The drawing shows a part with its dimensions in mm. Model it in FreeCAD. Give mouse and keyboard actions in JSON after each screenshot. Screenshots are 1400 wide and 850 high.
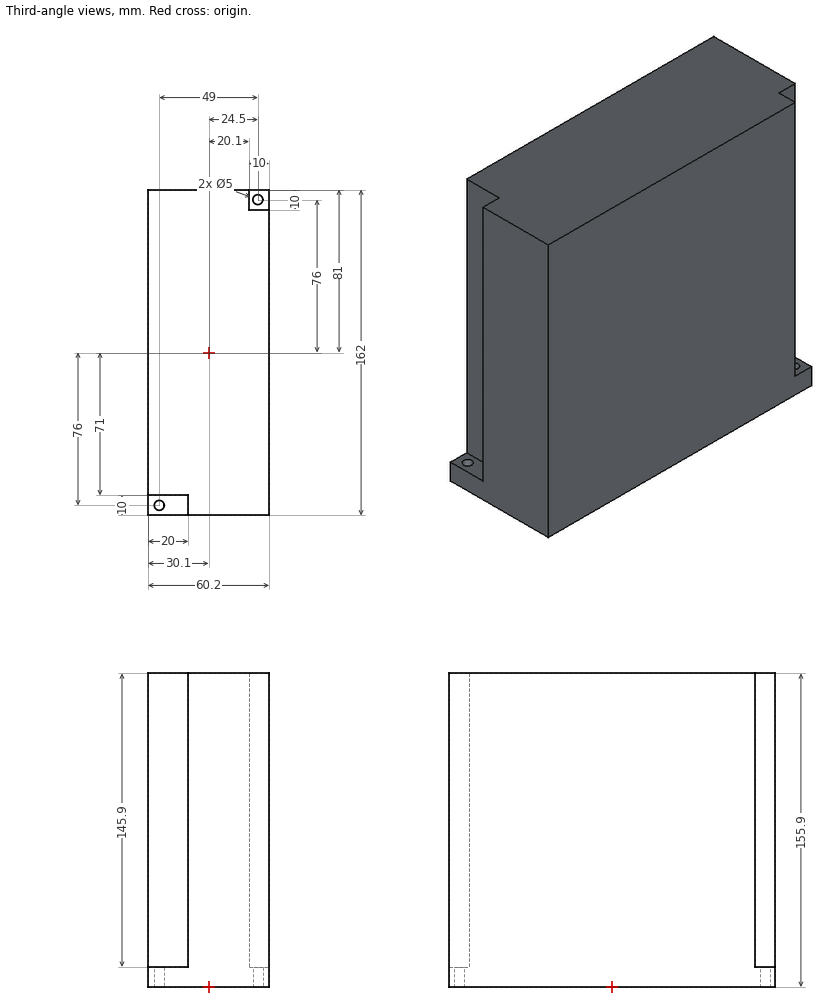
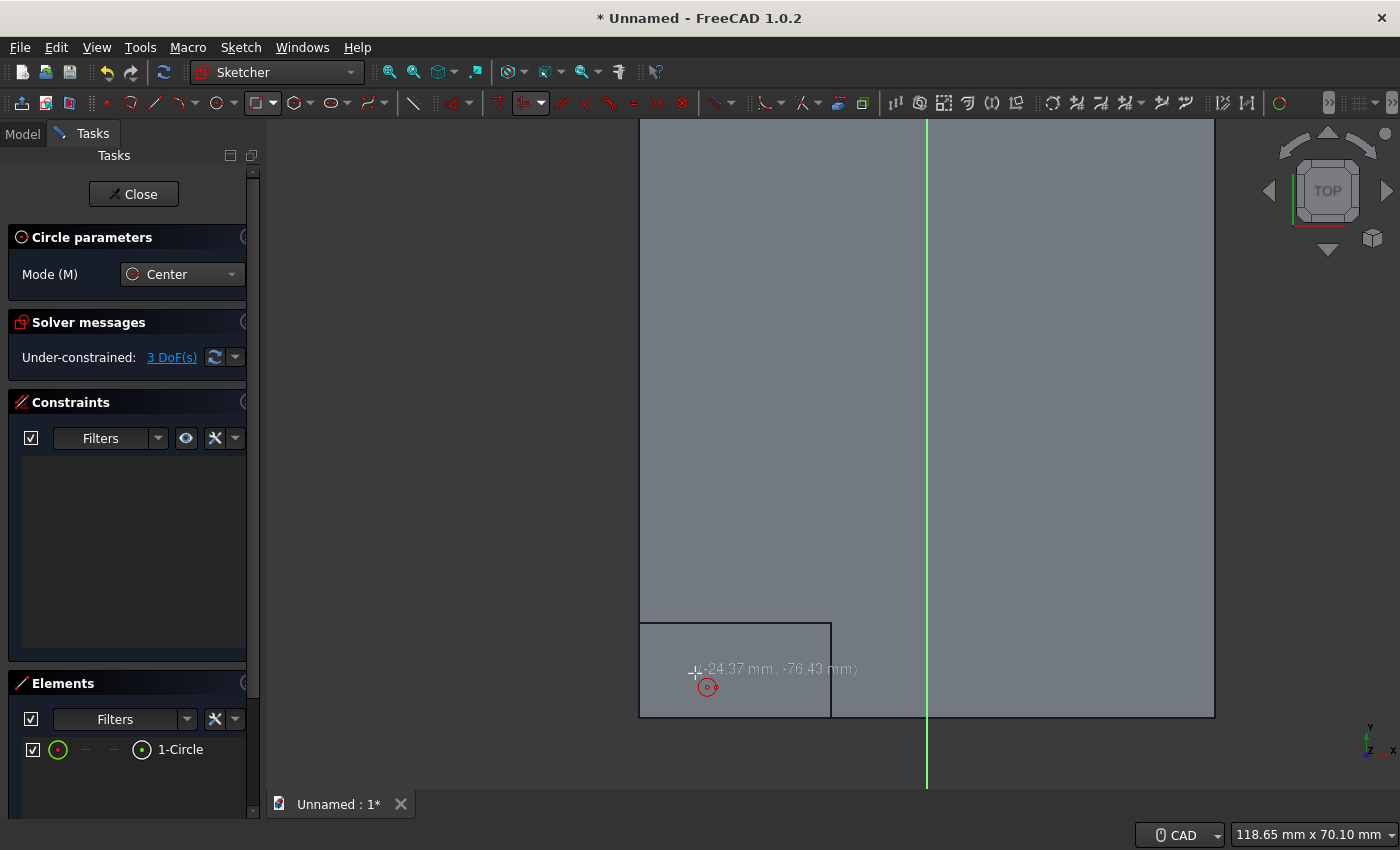
{"action": "left_click", "coordinate": [693, 670]}
{"action": "left_click", "coordinate": [710, 653]}
{"action": "key", "text": "Escape"}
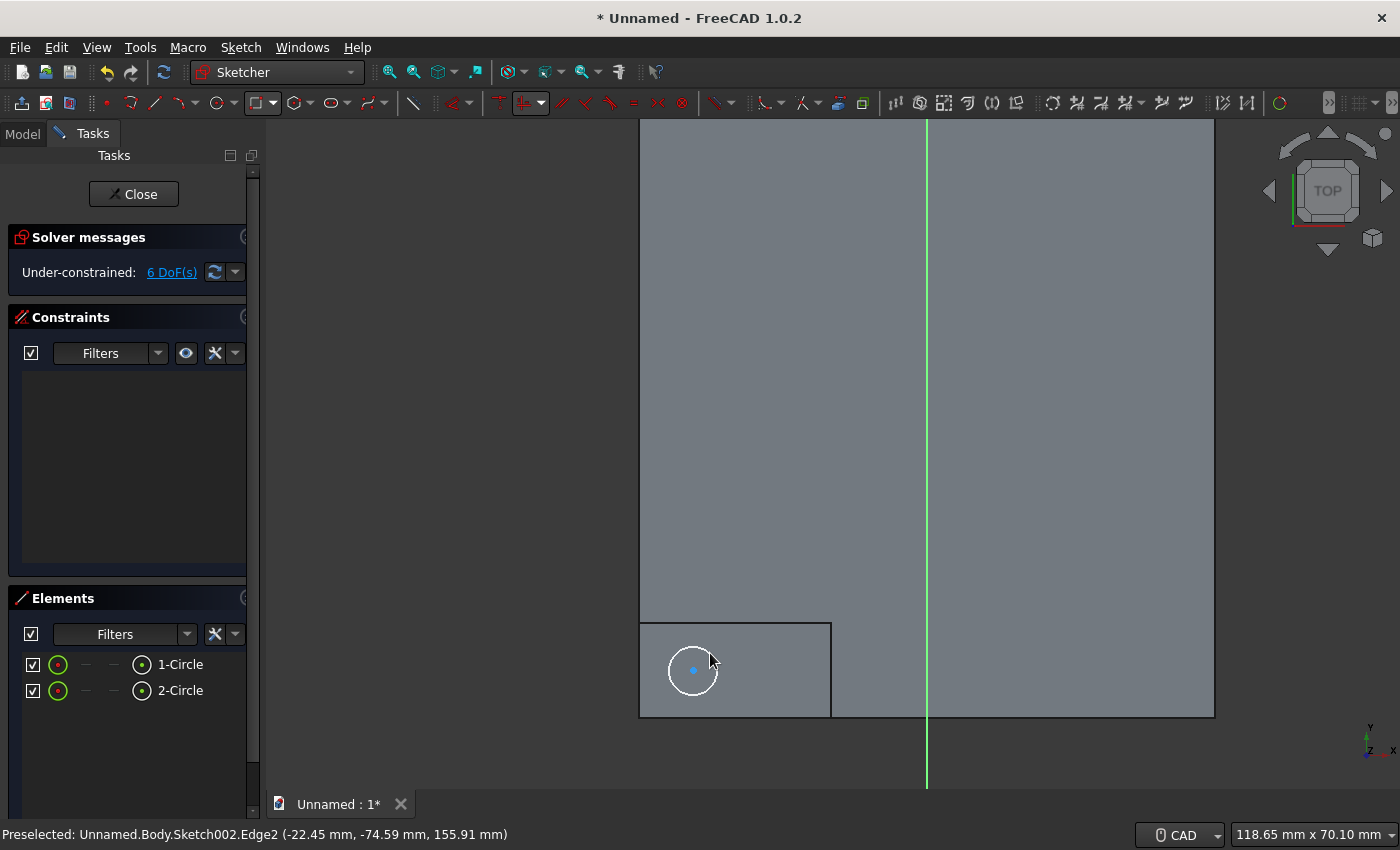
{"action": "scroll", "coordinate": [694, 674], "scroll_direction": "down", "scroll_amount": 6}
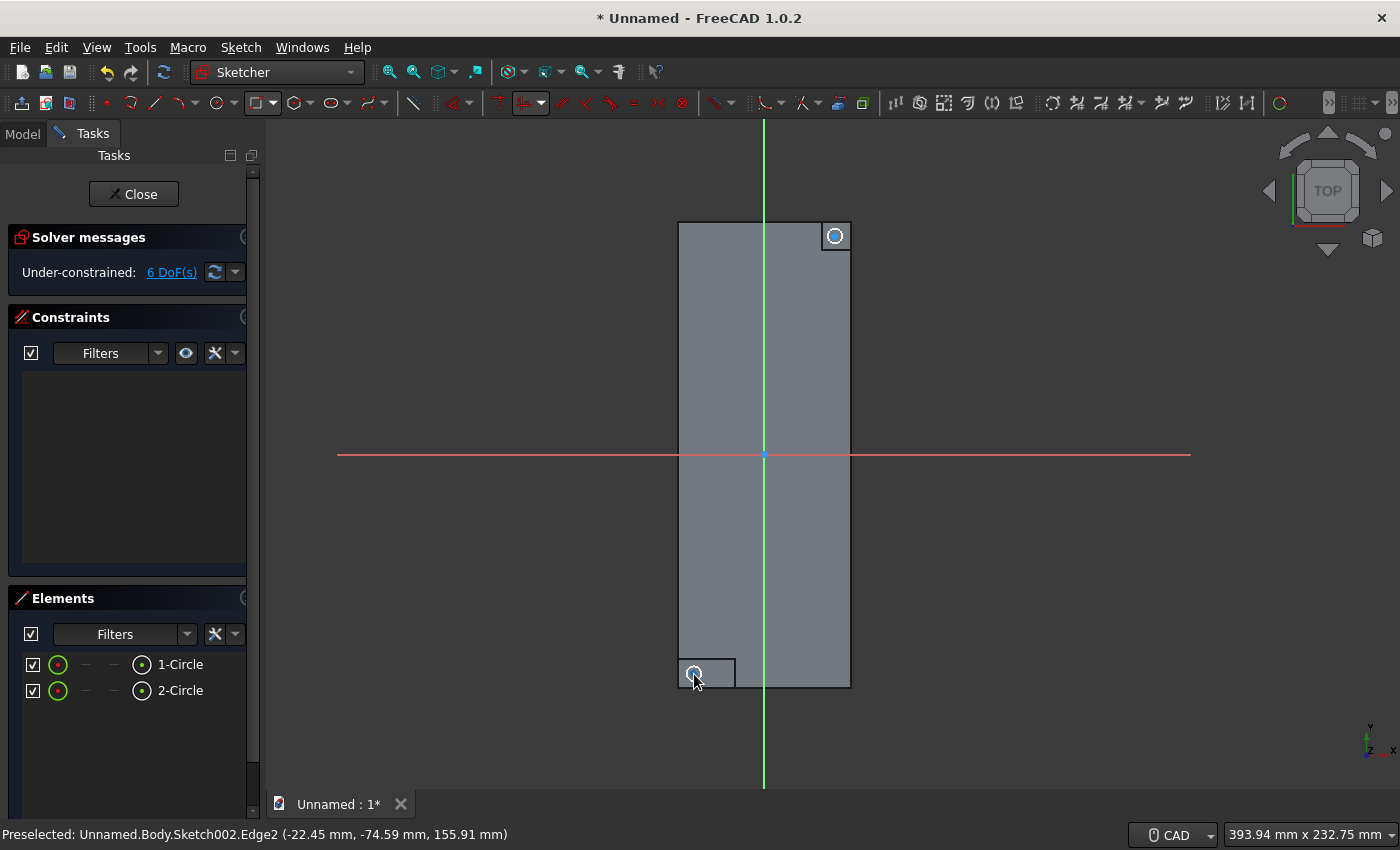
{"action": "scroll", "coordinate": [840, 231], "scroll_direction": "up", "scroll_amount": 4}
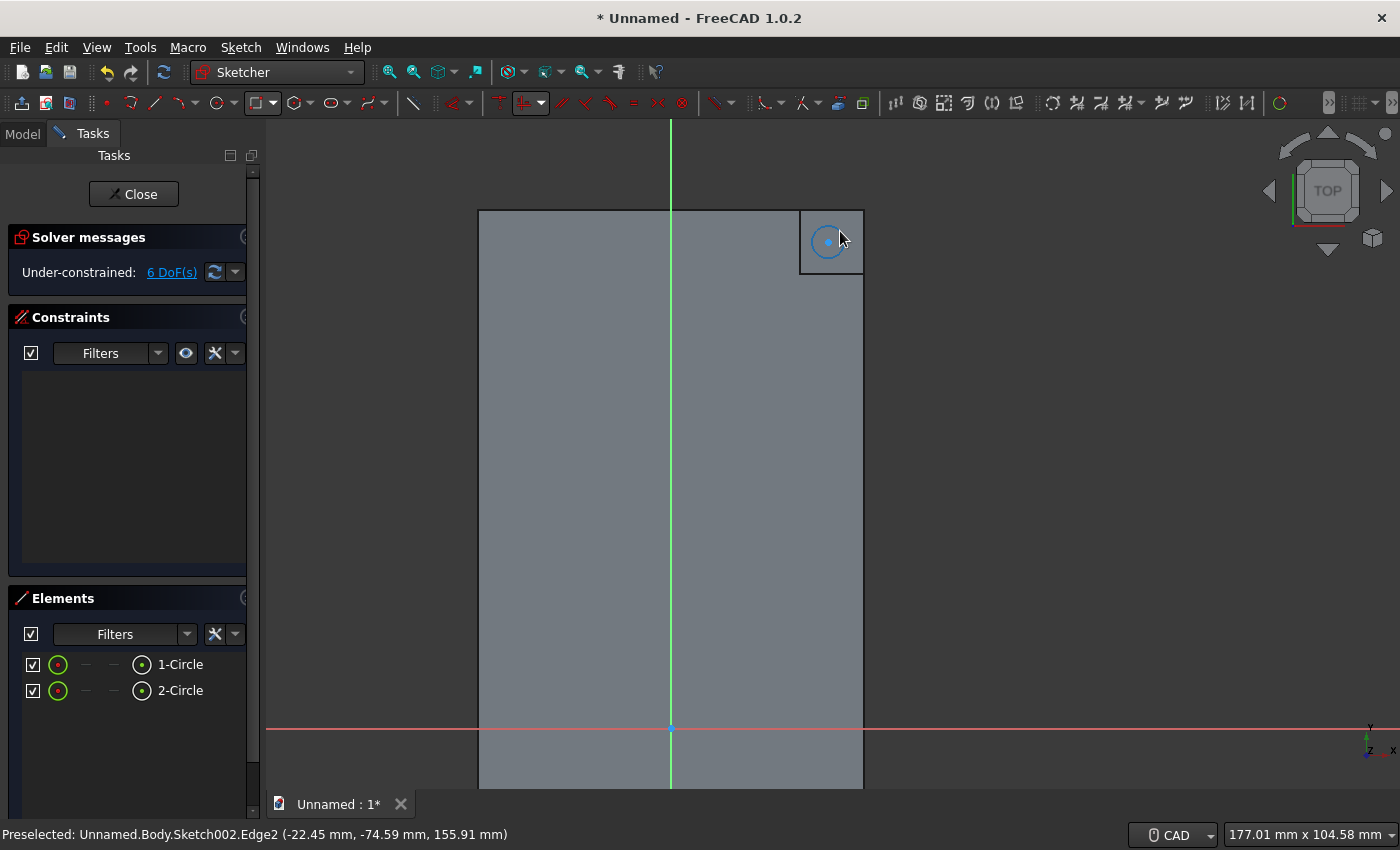
{"action": "left_click", "coordinate": [839, 231]}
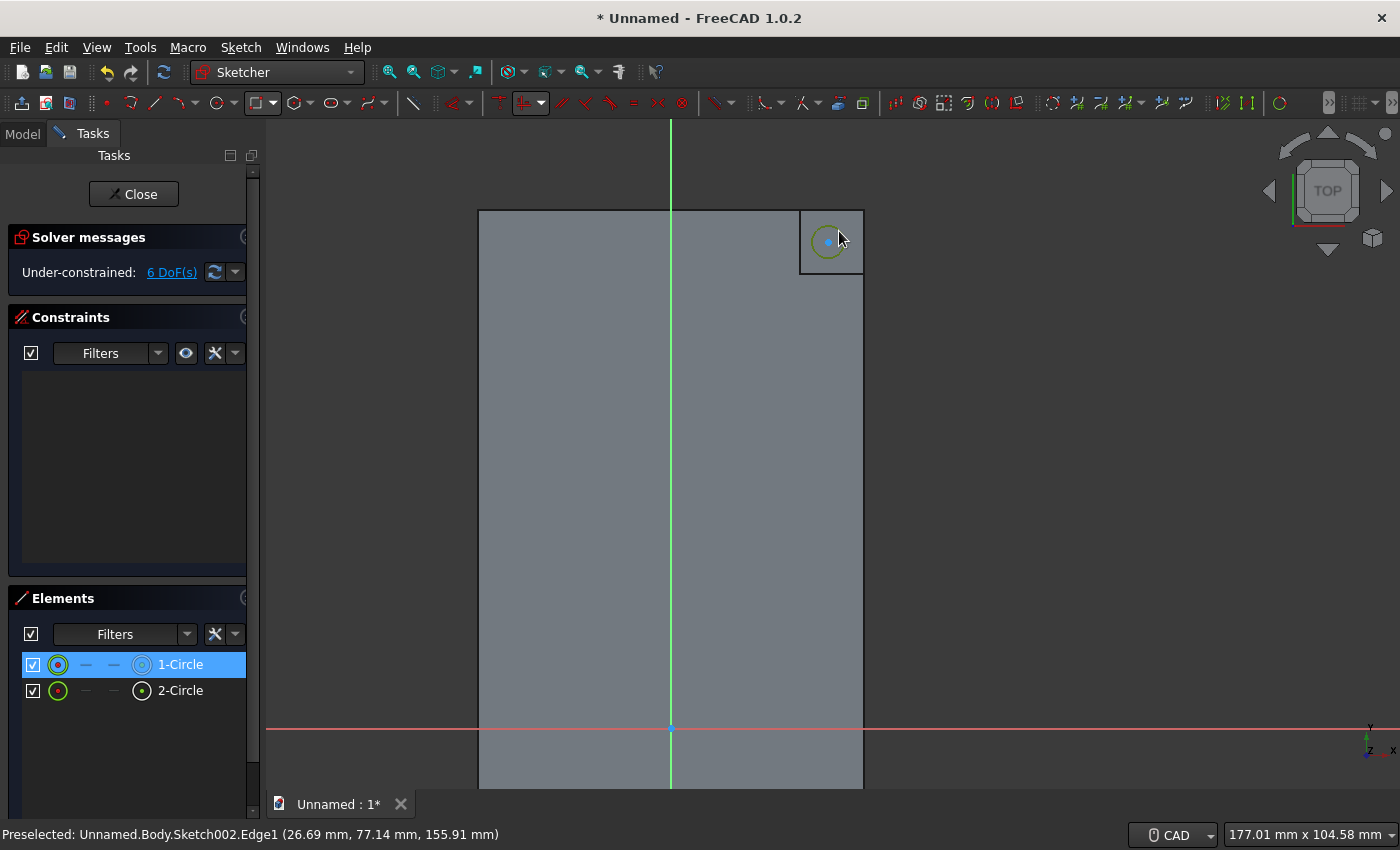
{"action": "scroll", "coordinate": [841, 230], "scroll_direction": "down", "scroll_amount": 4}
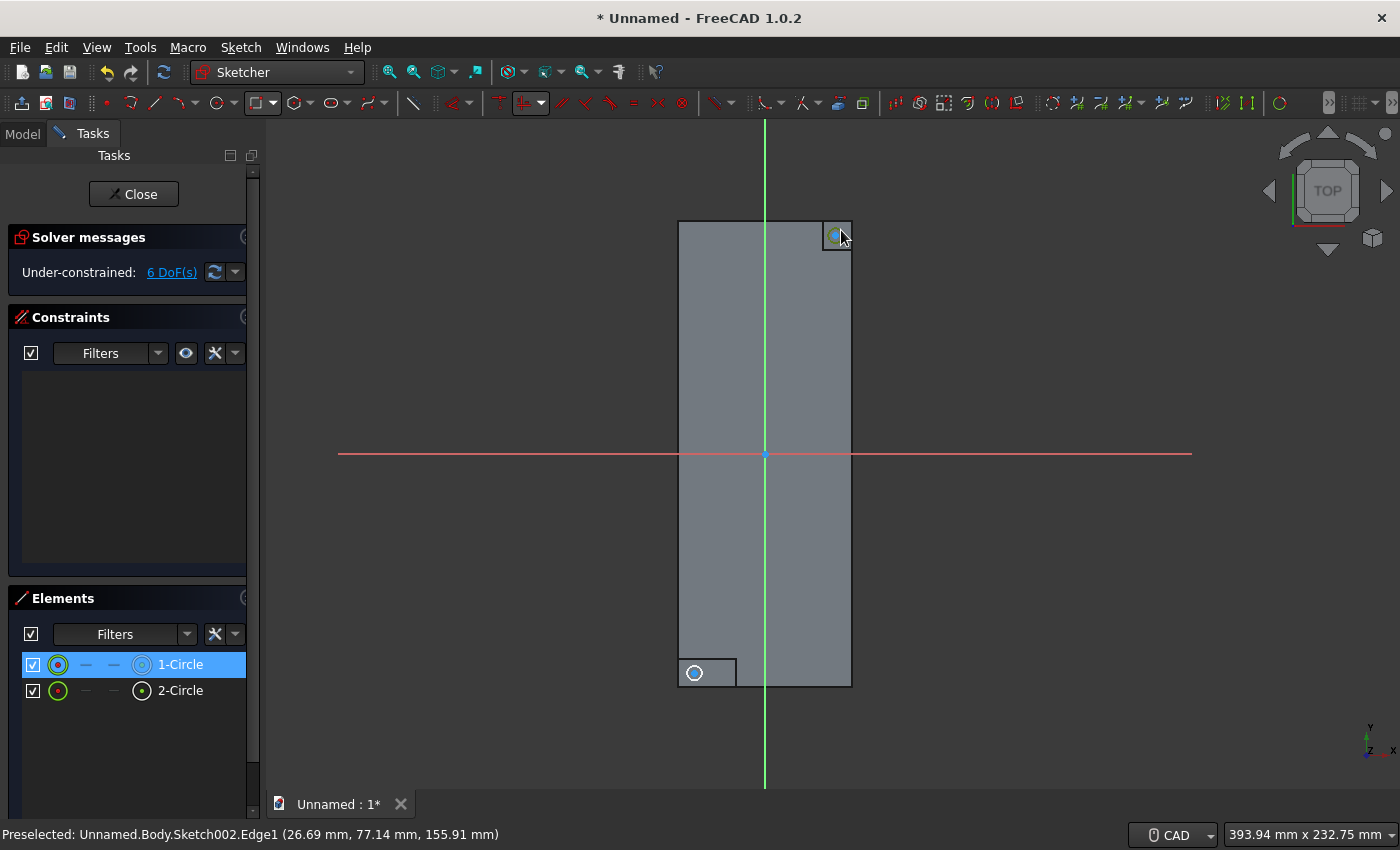
{"action": "scroll", "coordinate": [700, 668], "scroll_direction": "up", "scroll_amount": 4}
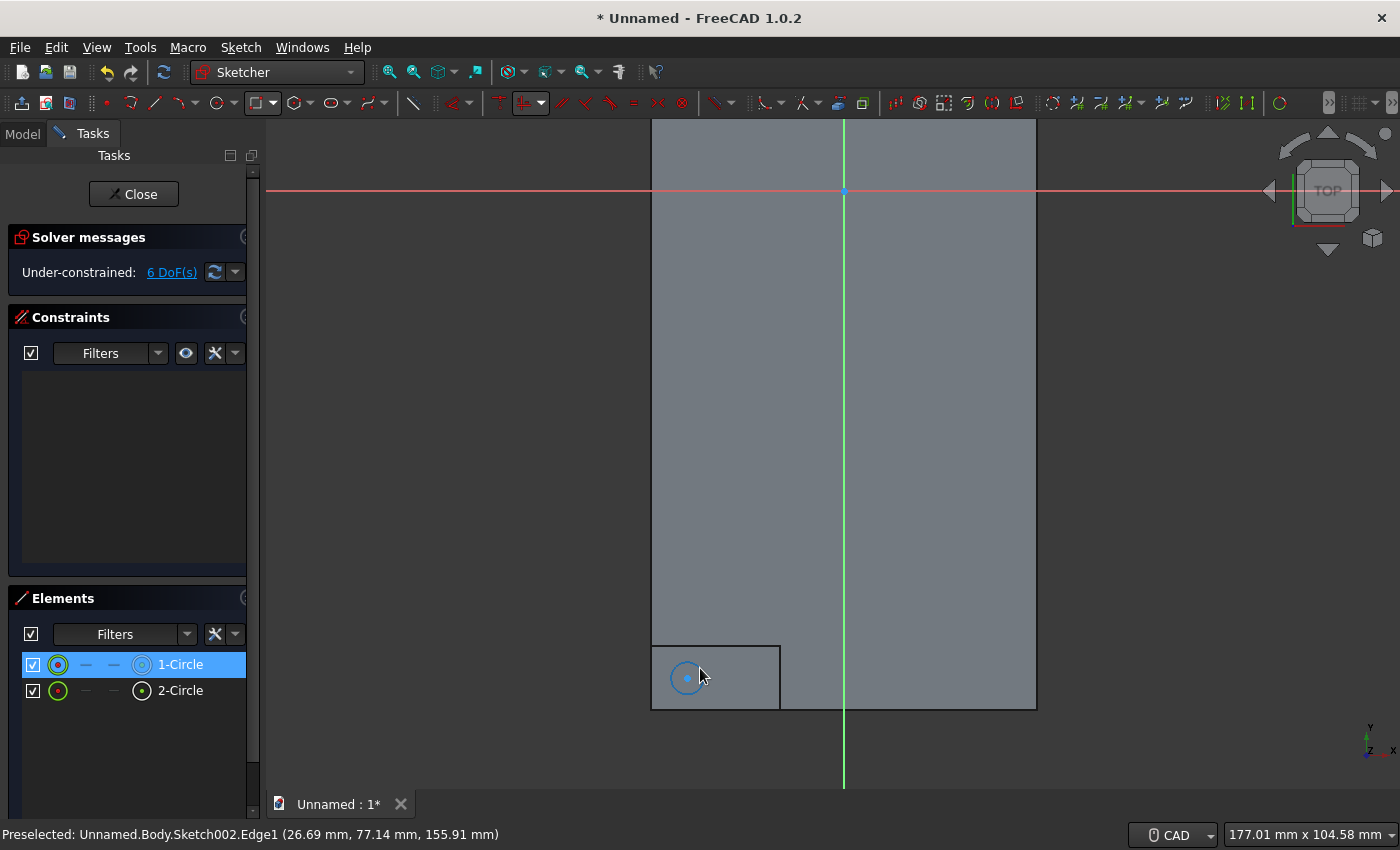
{"action": "left_click", "coordinate": [699, 667]}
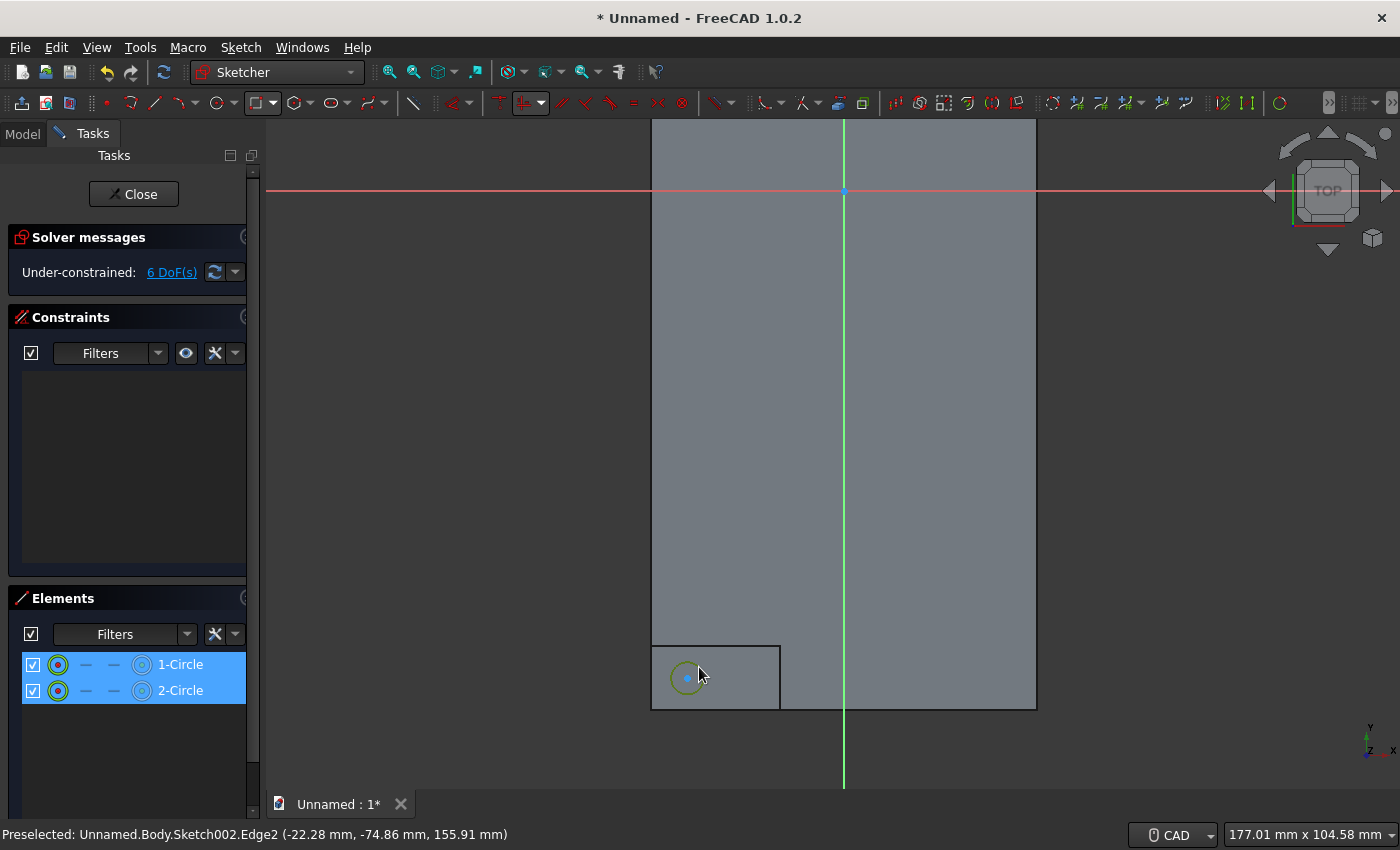
{"action": "key", "text": "e"}